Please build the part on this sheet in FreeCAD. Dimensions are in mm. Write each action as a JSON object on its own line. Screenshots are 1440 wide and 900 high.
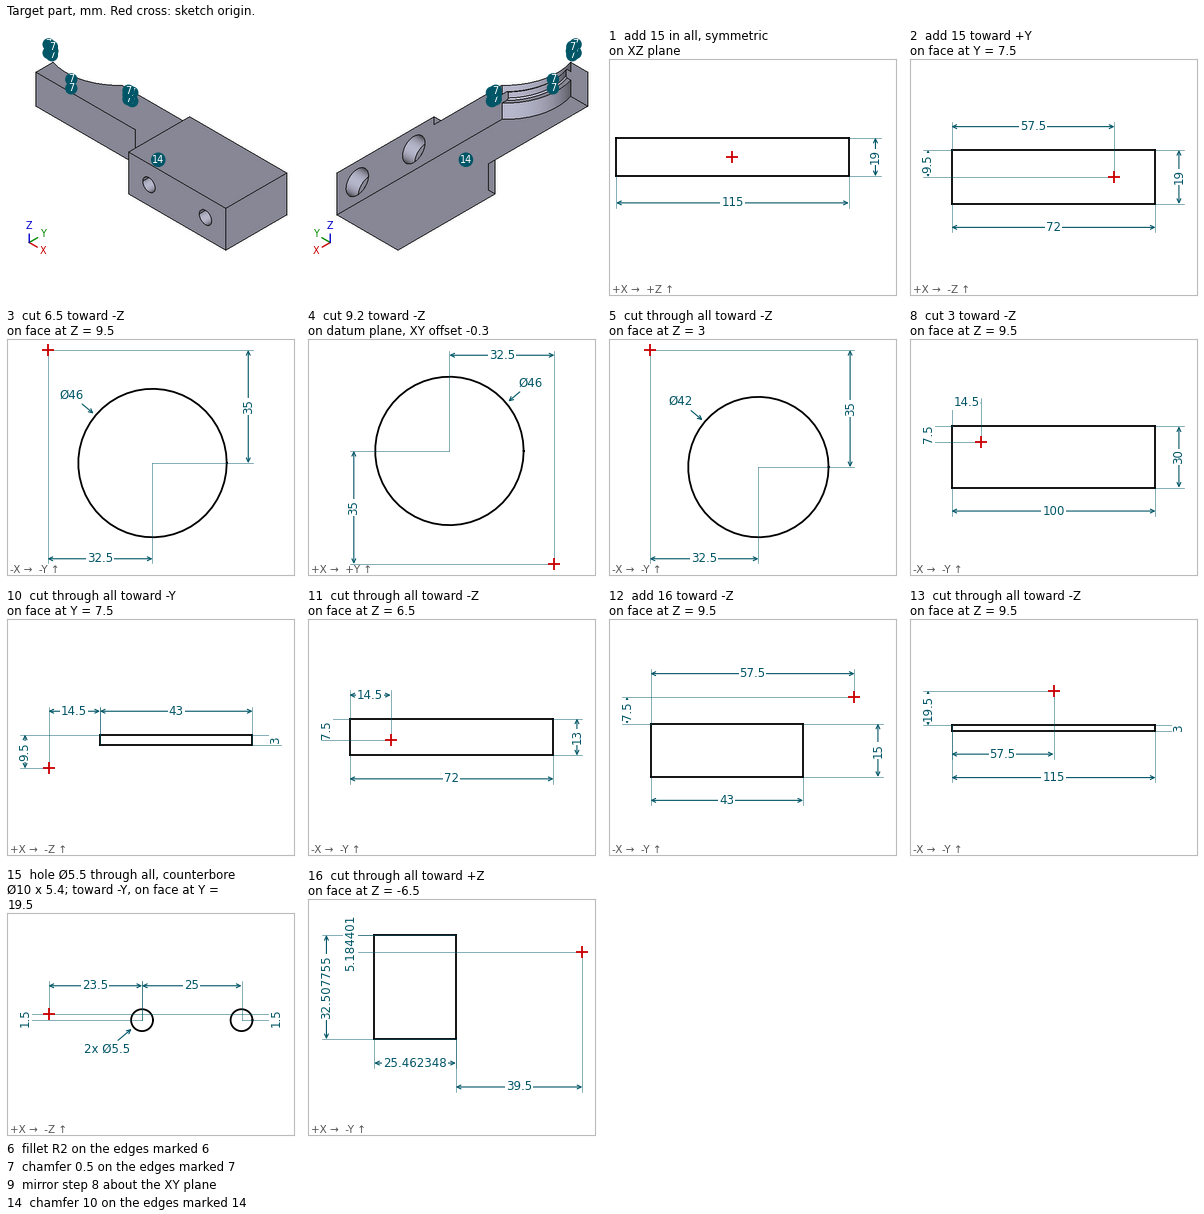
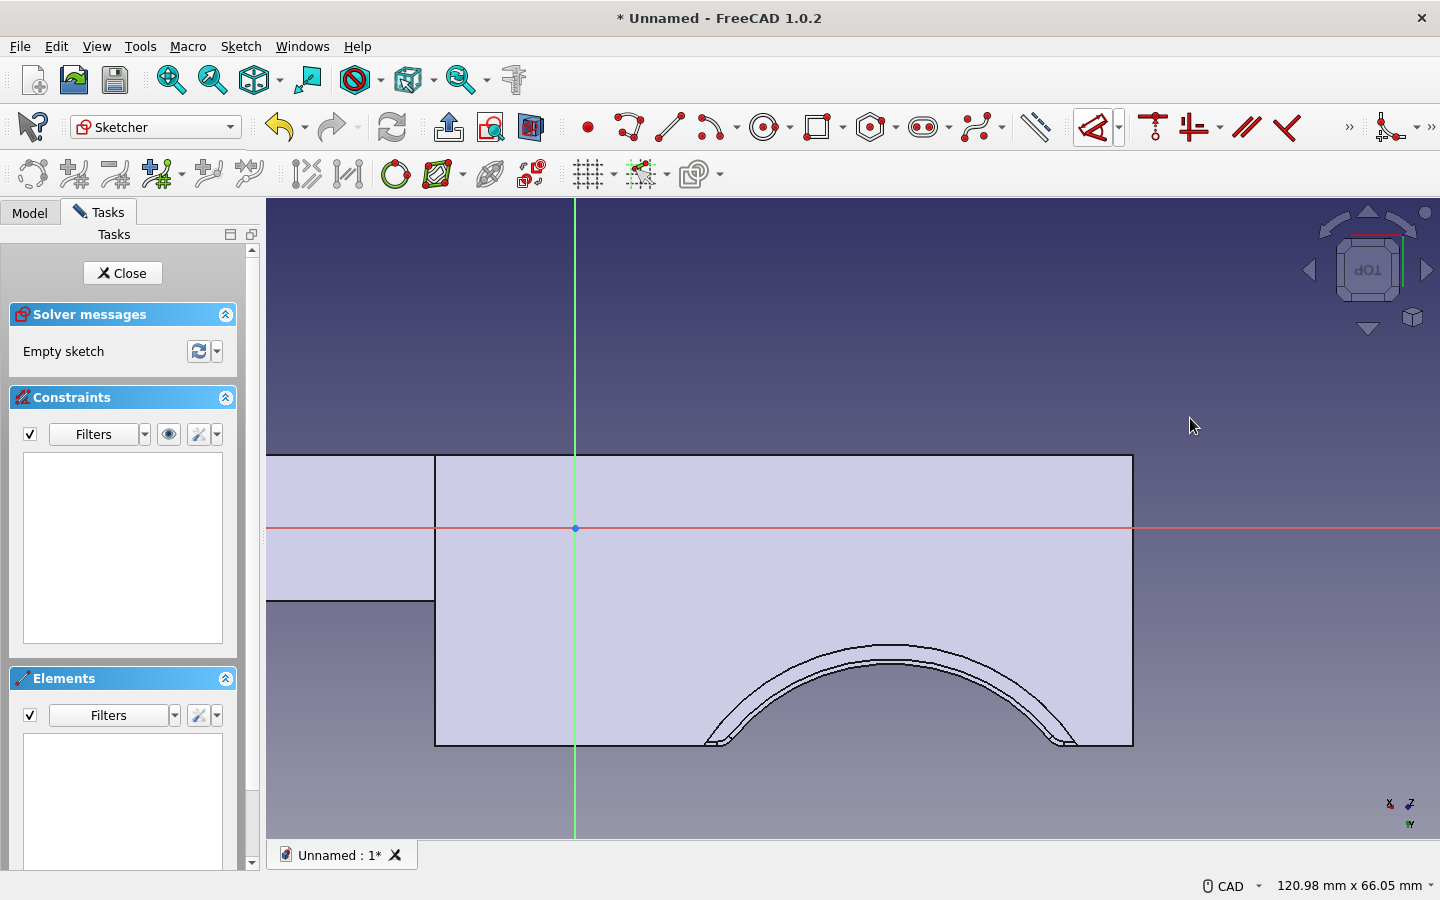
{"action": "left_click", "coordinate": [816, 128]}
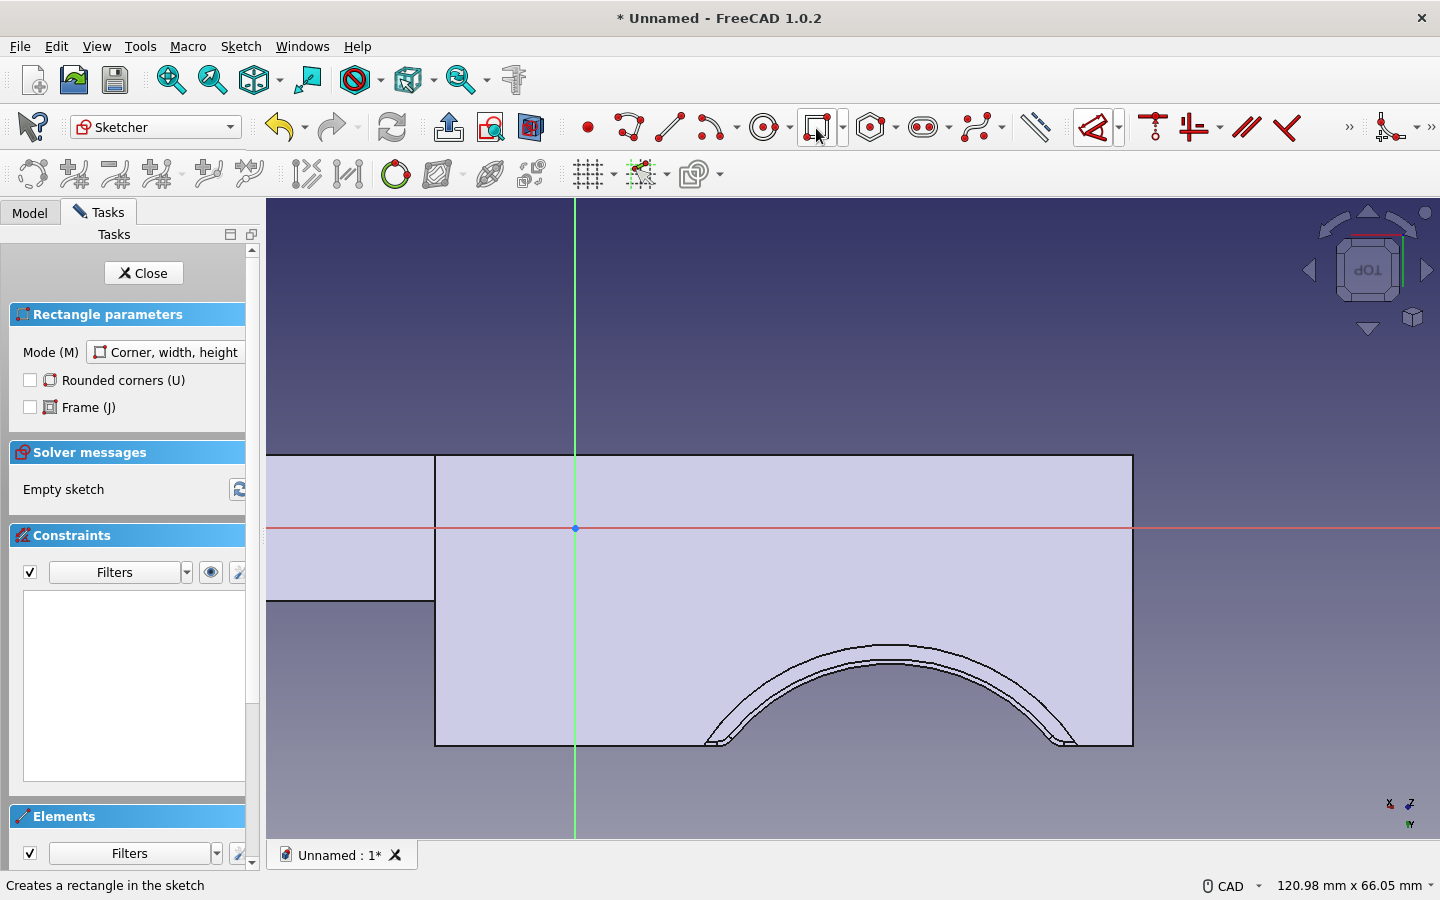
{"action": "left_click", "coordinate": [435, 455]}
{"action": "mouse_move", "coordinate": [1133, 581]}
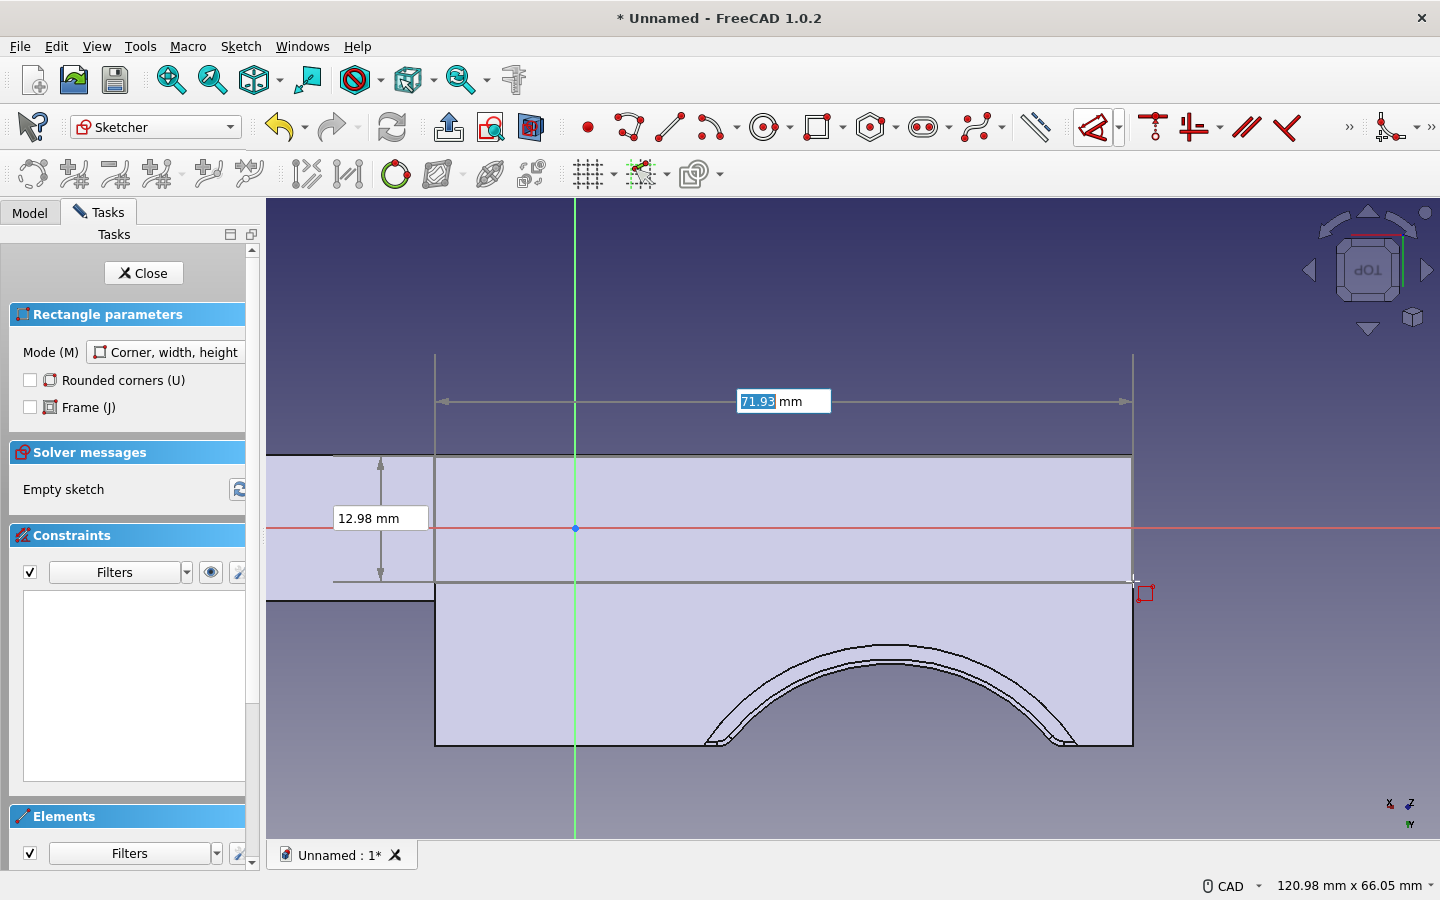
{"action": "type", "text": "72"}
{"action": "key", "text": "Tab"}
{"action": "type", "text": "13"}
{"action": "key", "text": "Return"}
{"action": "key", "text": "Escape"}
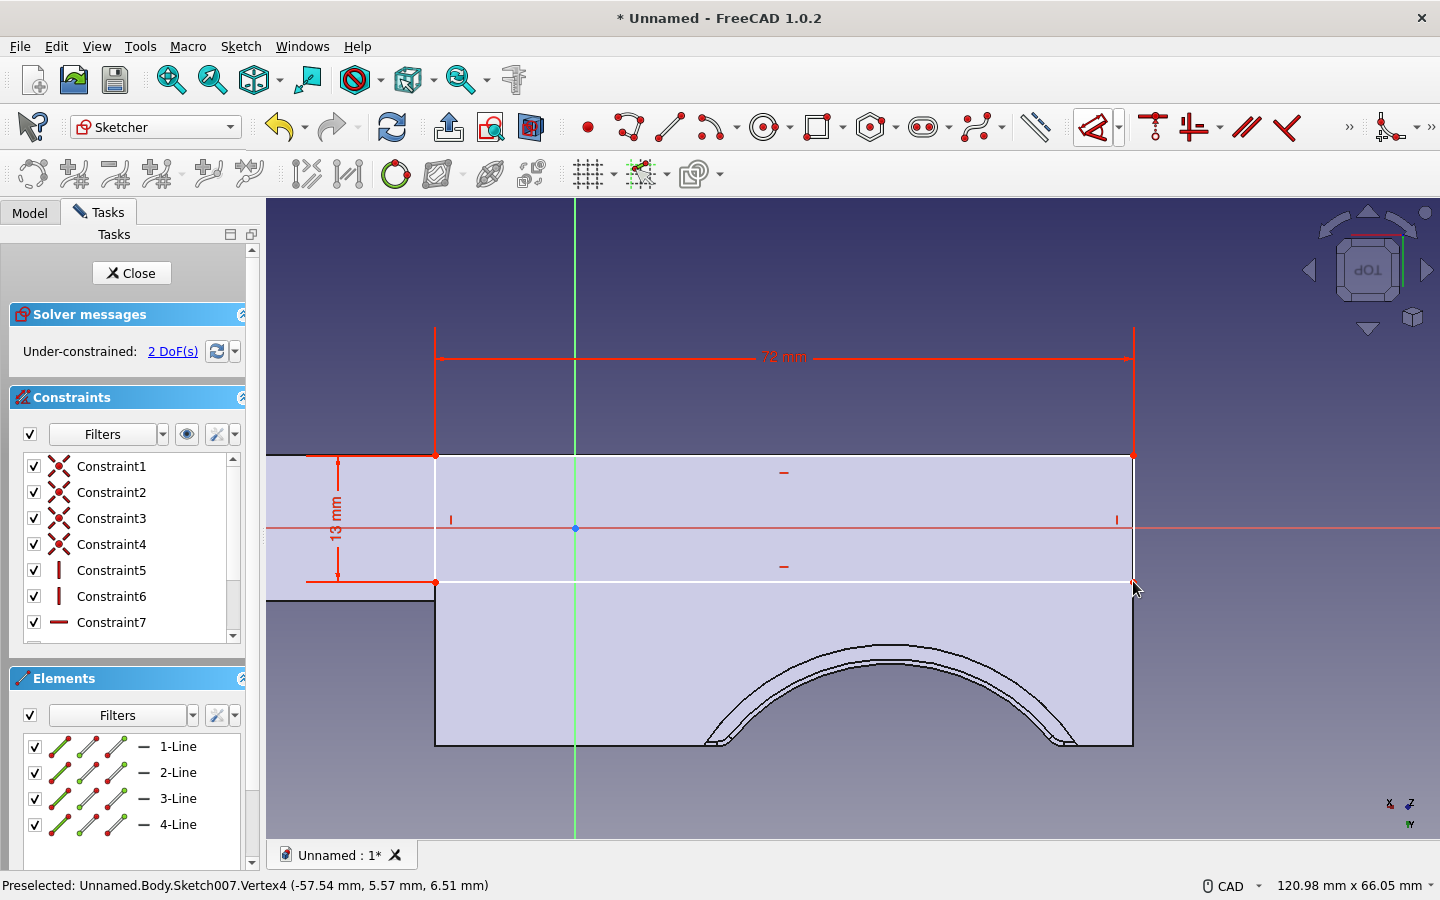
{"action": "left_click", "coordinate": [435, 456]}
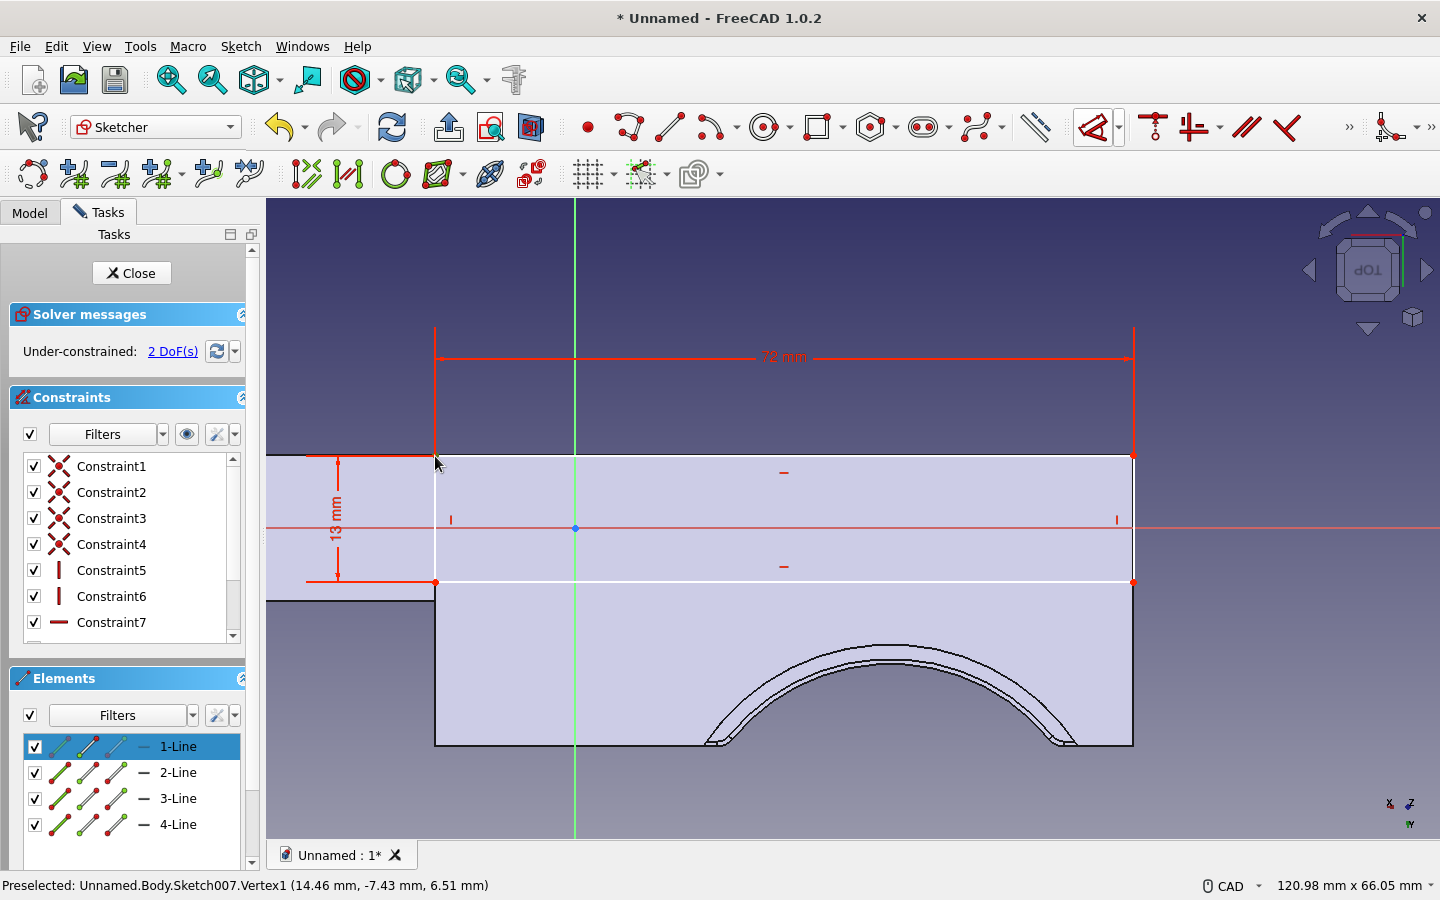
{"action": "key", "text": "i"}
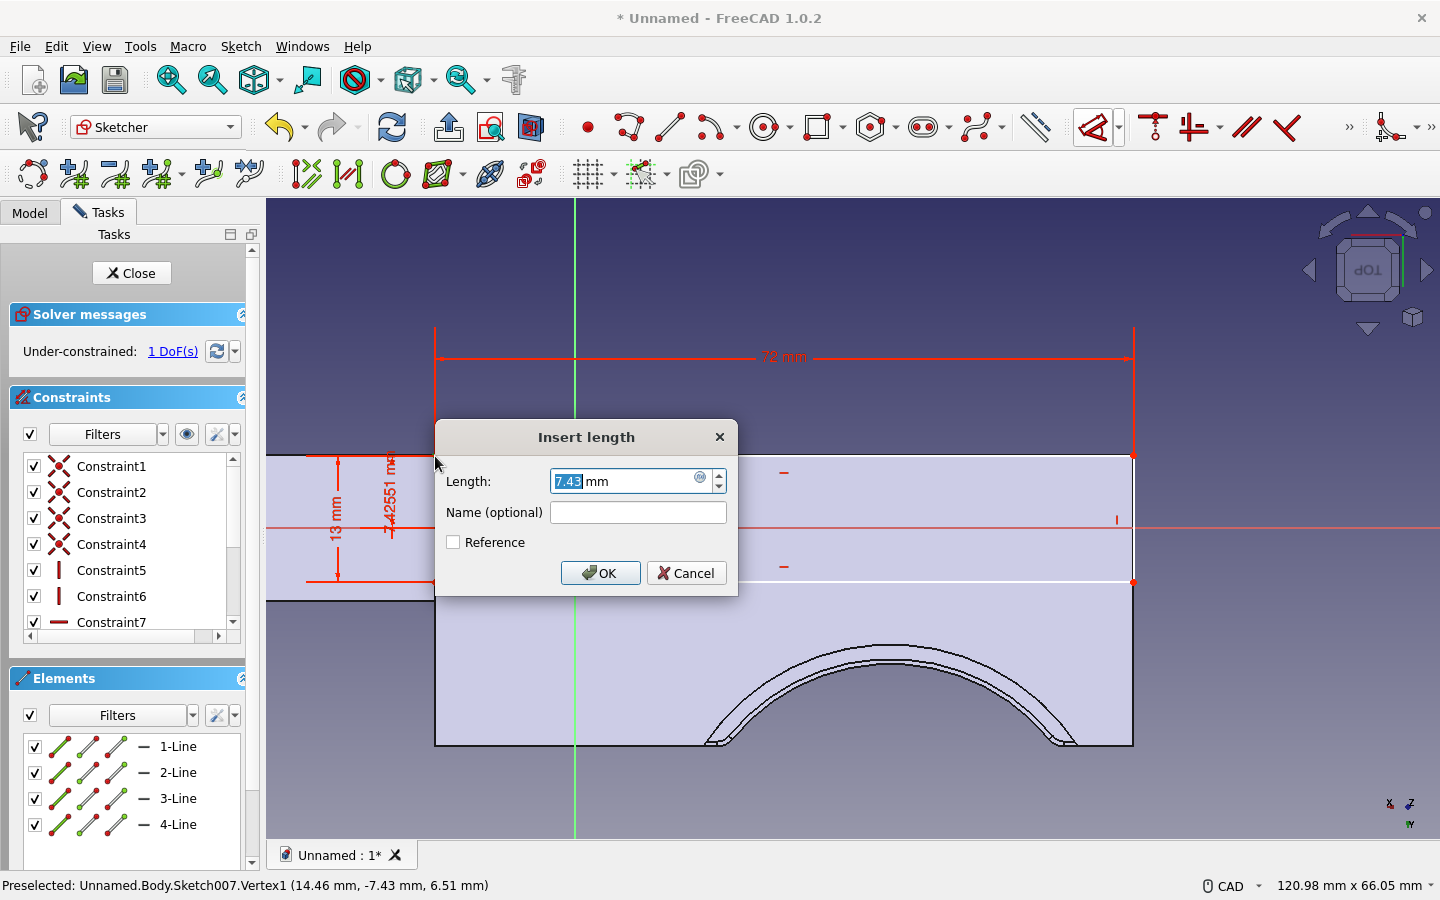
{"action": "type", "text": "7.5"}
{"action": "key", "text": "Return"}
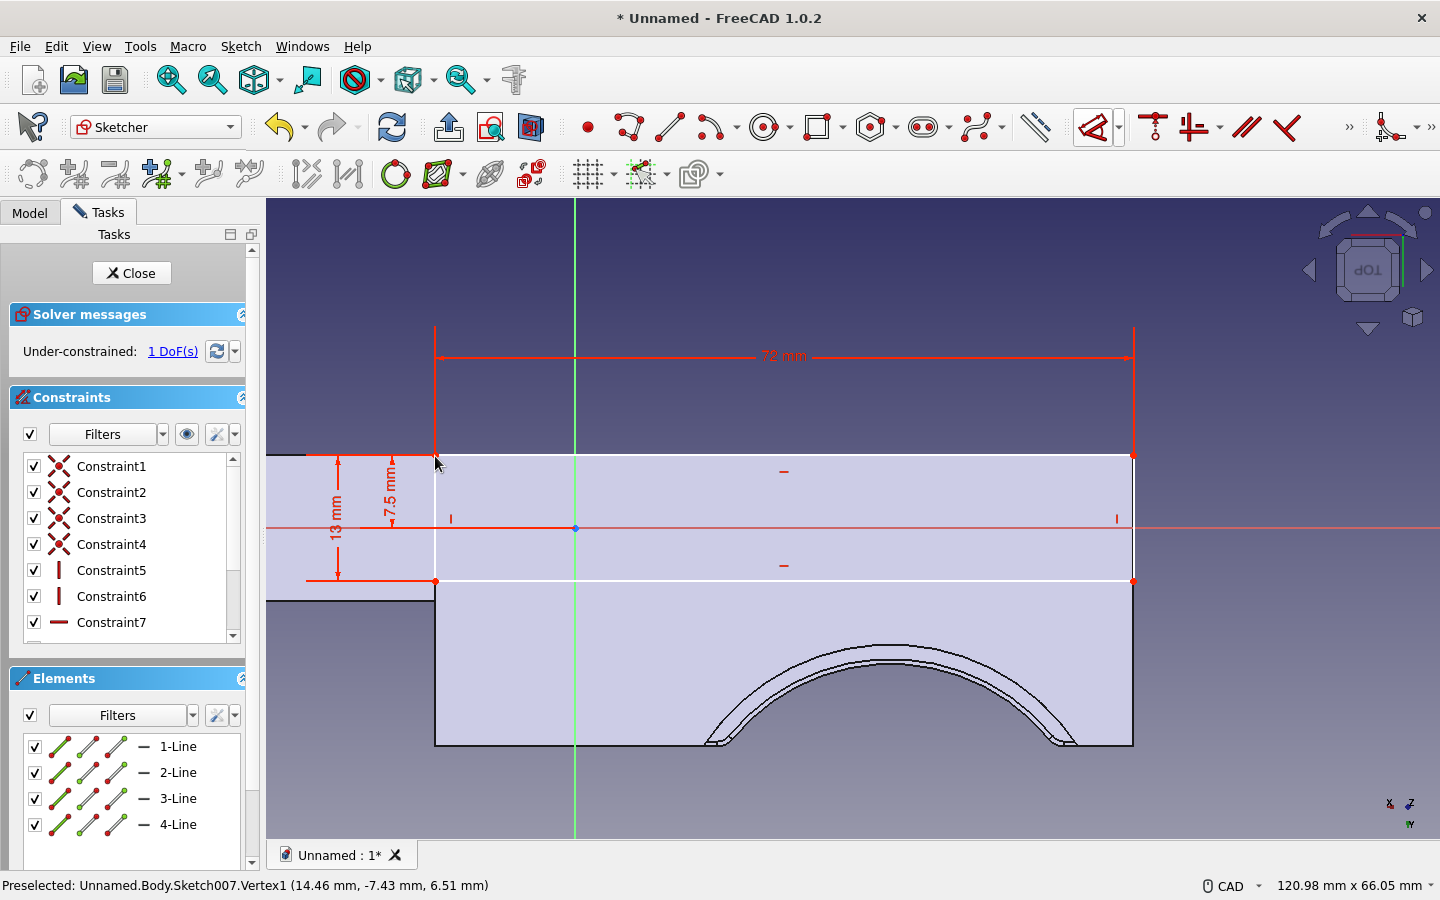
{"action": "left_click", "coordinate": [435, 455]}